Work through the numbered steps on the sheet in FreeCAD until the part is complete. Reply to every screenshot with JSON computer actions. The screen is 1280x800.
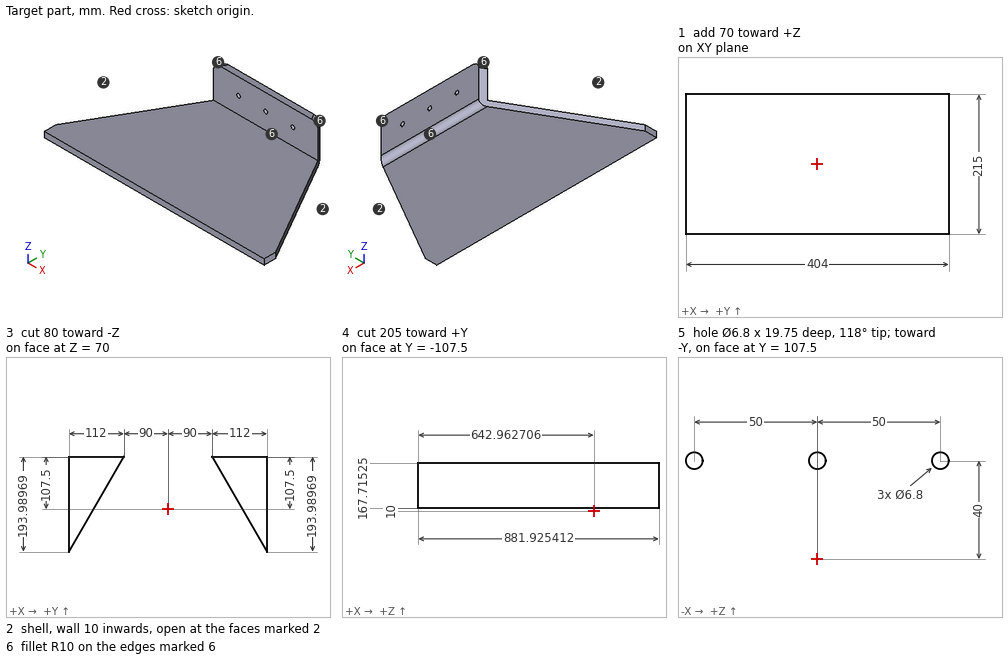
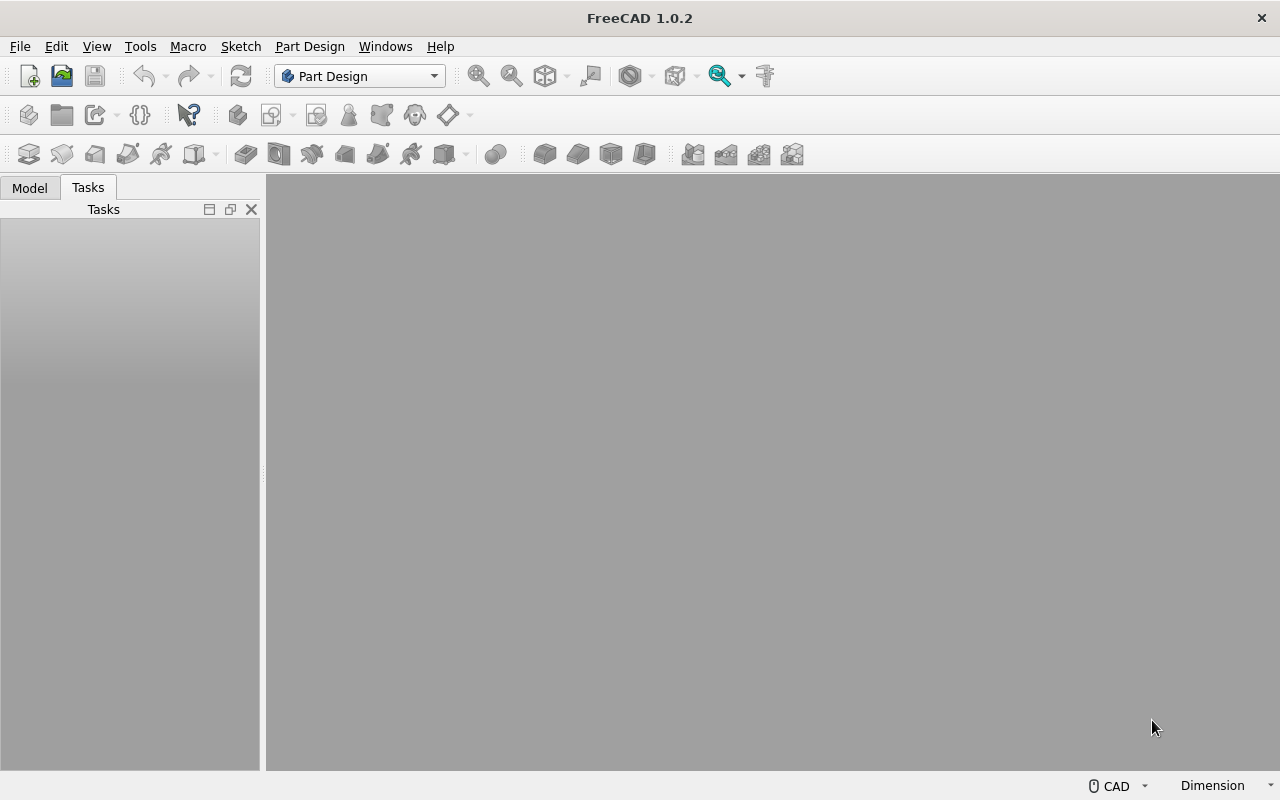
{"action": "left_click", "coordinate": [29, 76]}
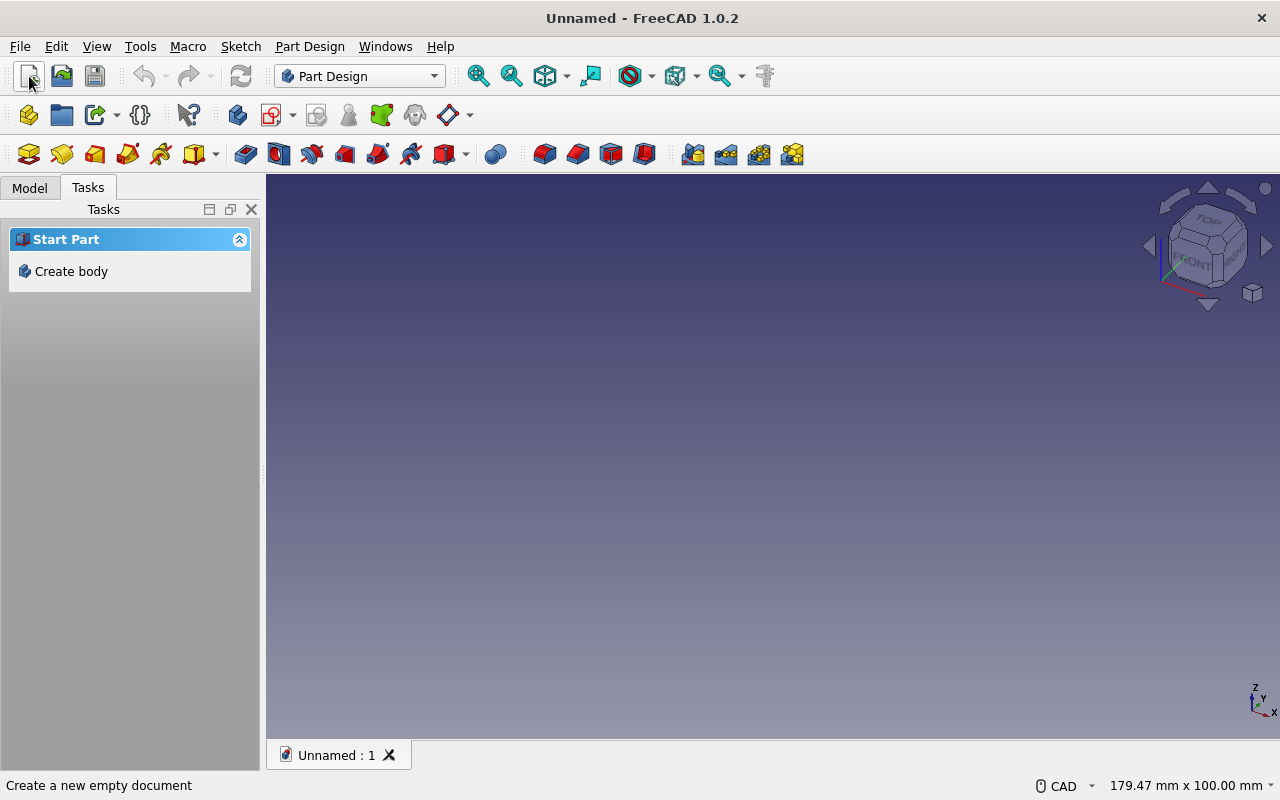
{"action": "left_click", "coordinate": [270, 116]}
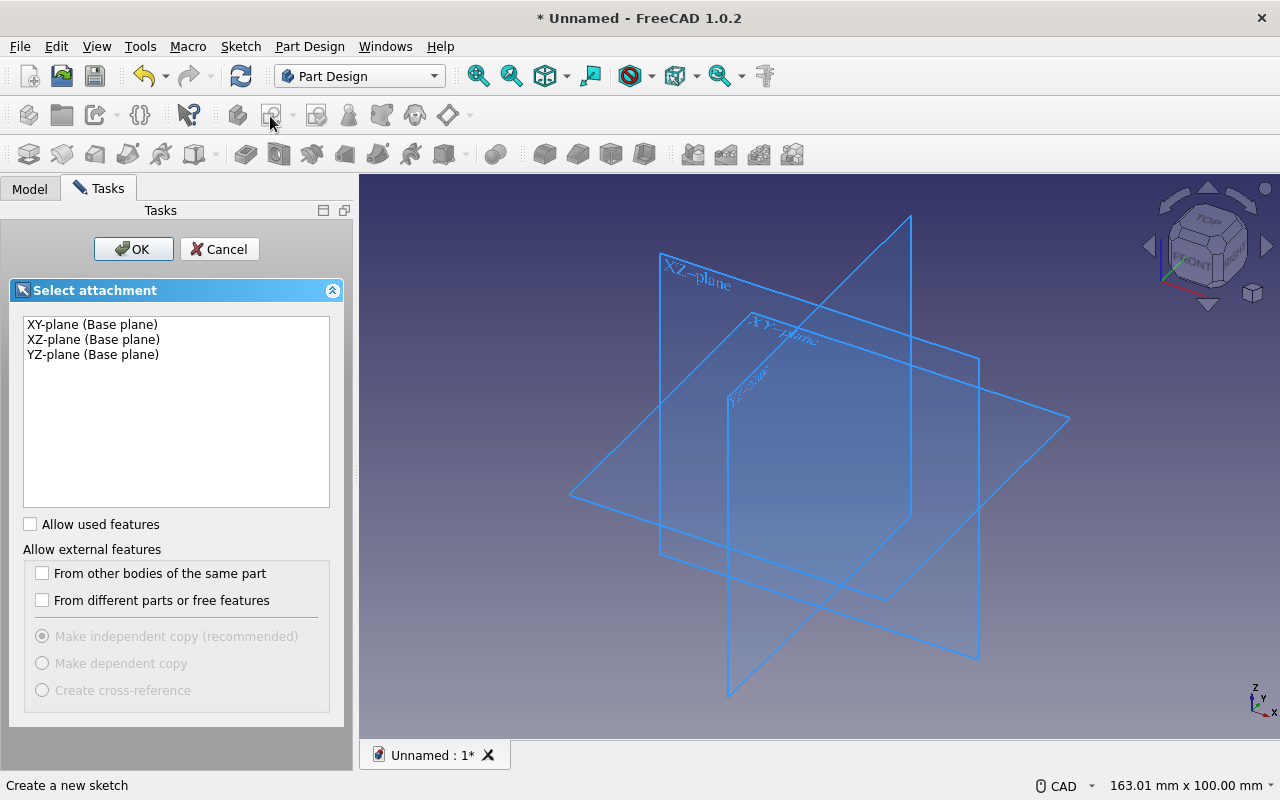
{"action": "left_click", "coordinate": [84, 324]}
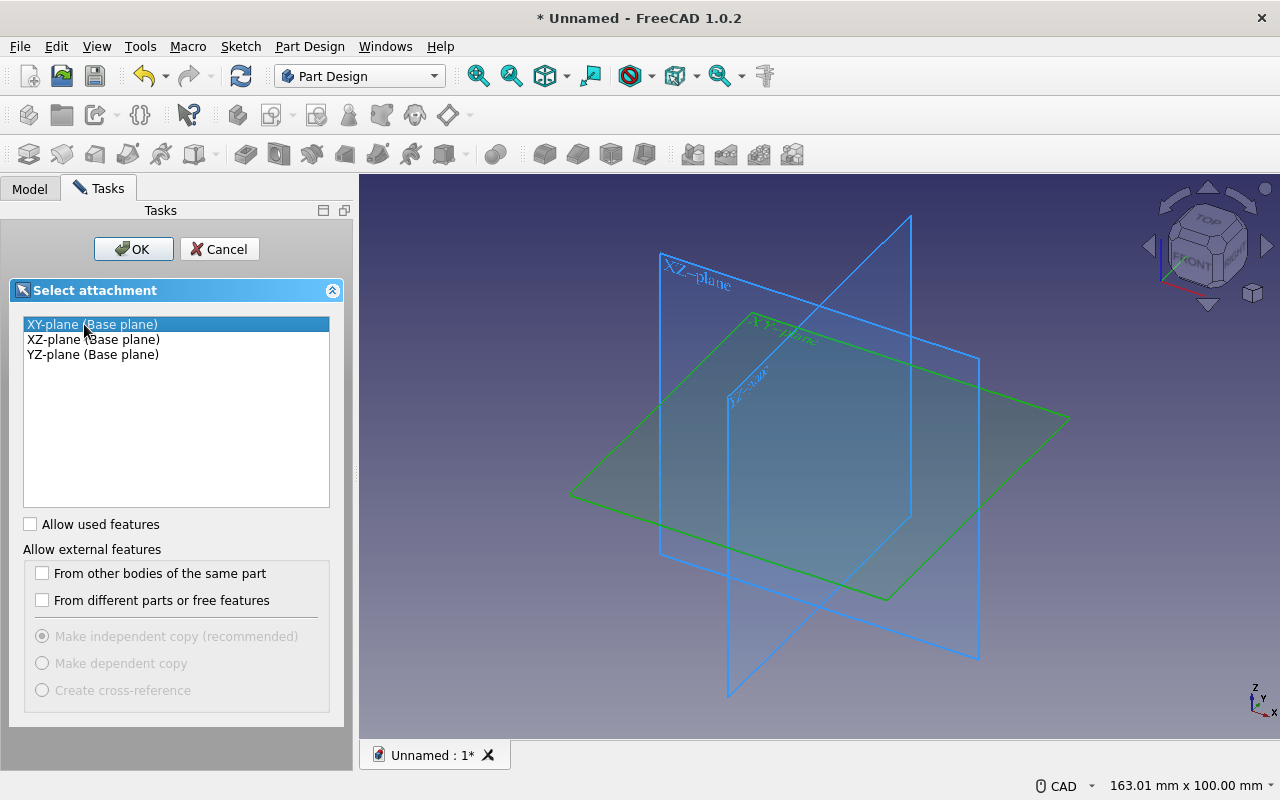
{"action": "left_click", "coordinate": [134, 249]}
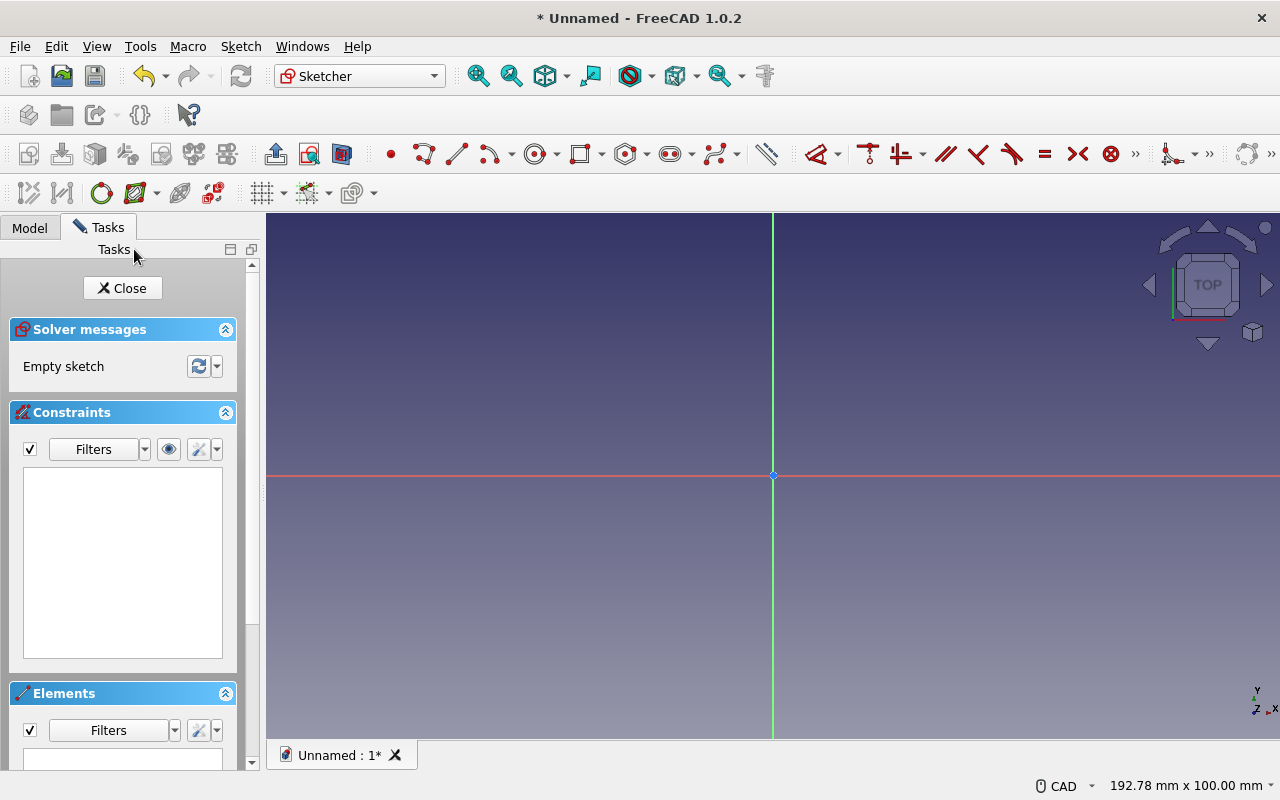
{"action": "scroll", "coordinate": [675, 476], "scroll_direction": "down", "scroll_amount": 6}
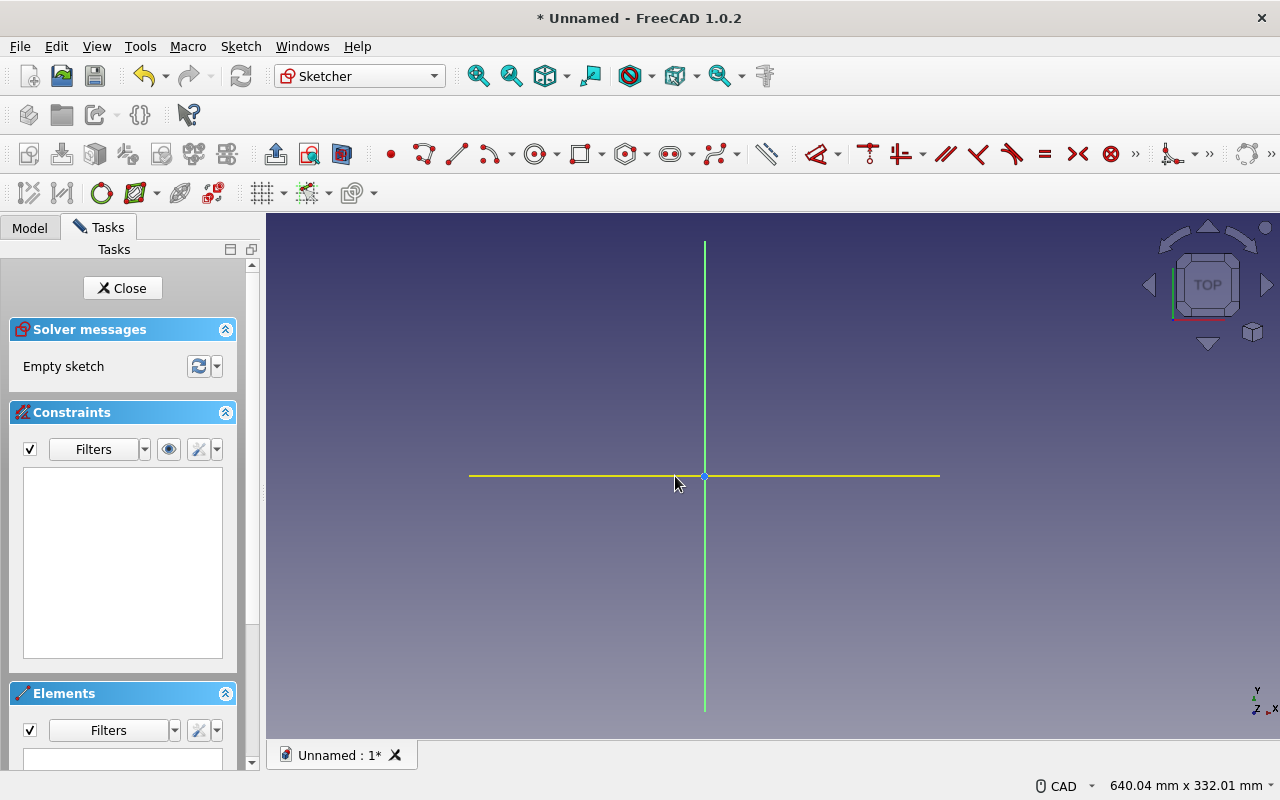
{"action": "key", "text": "g v"}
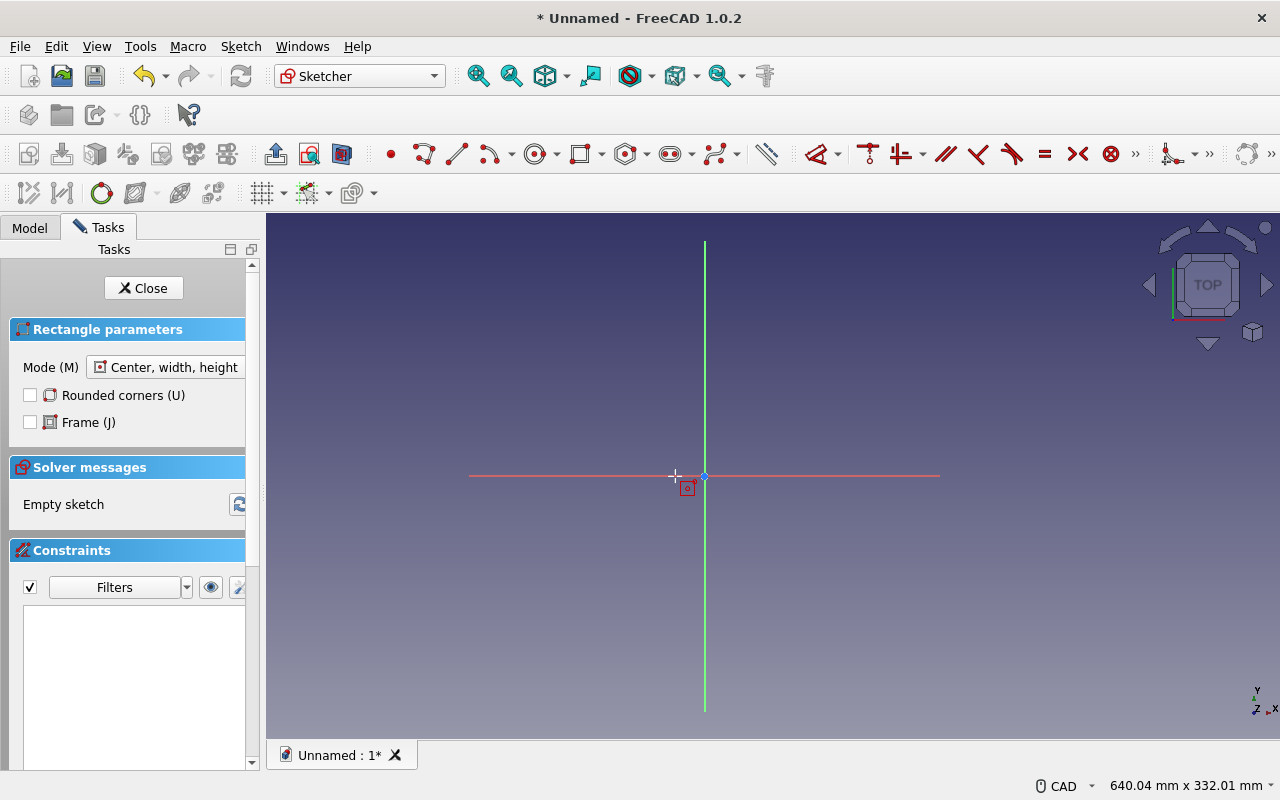
{"action": "left_click", "coordinate": [705, 476]}
{"action": "left_click", "coordinate": [1025, 306]}
{"action": "key", "text": "Escape"}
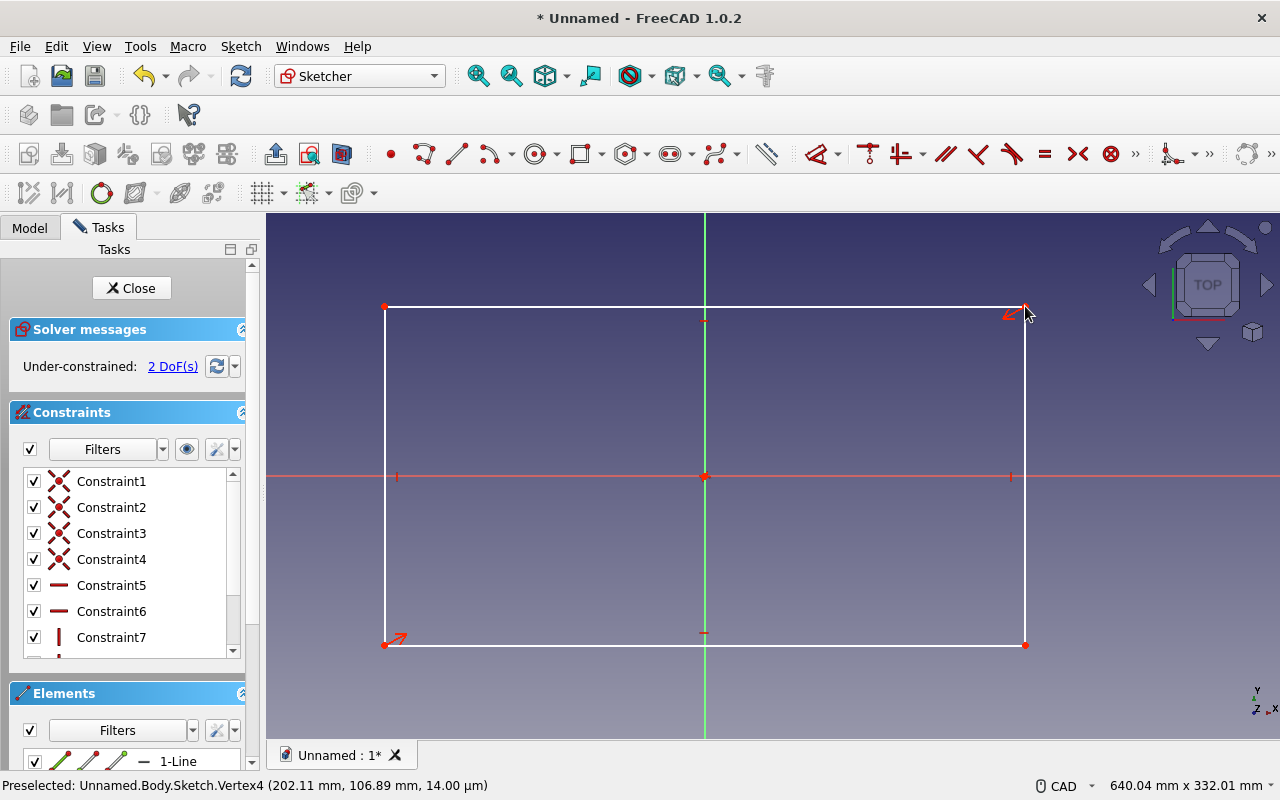
{"action": "left_click", "coordinate": [577, 646]}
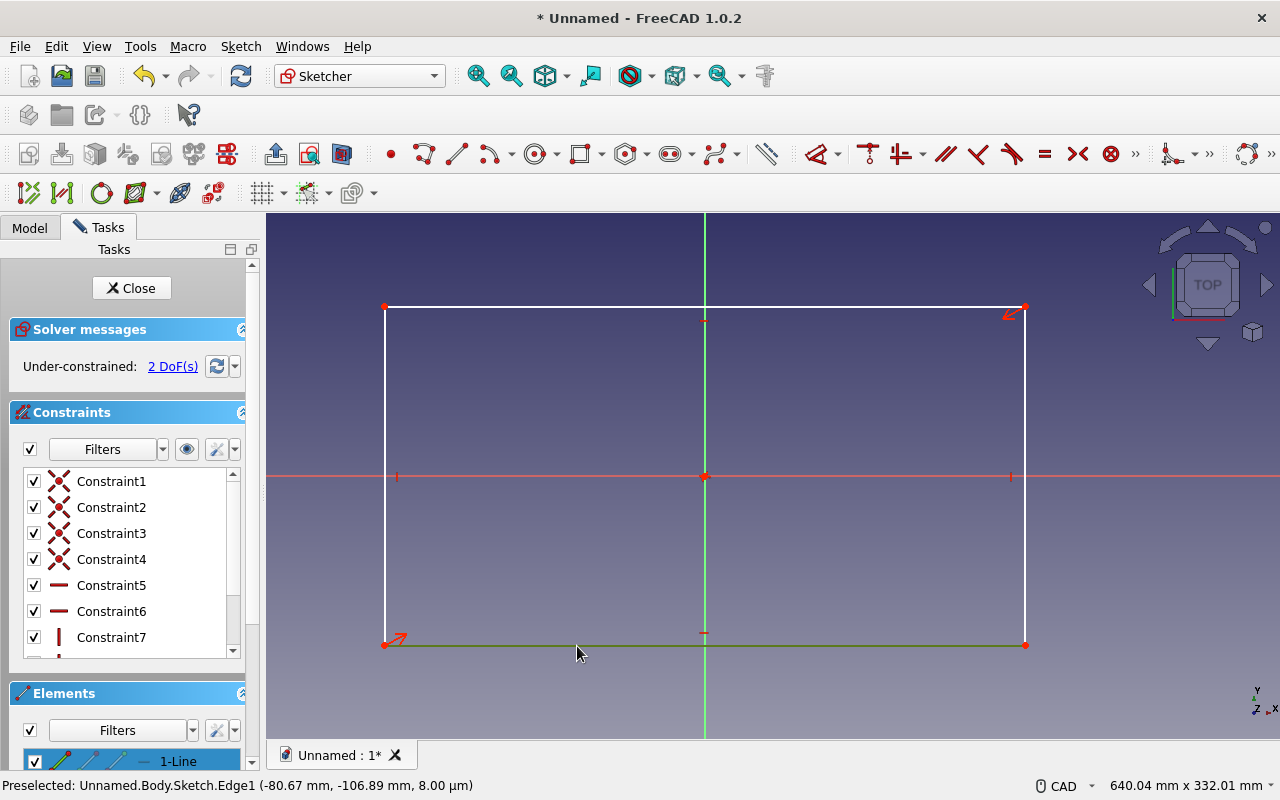
{"action": "left_click", "coordinate": [838, 154]}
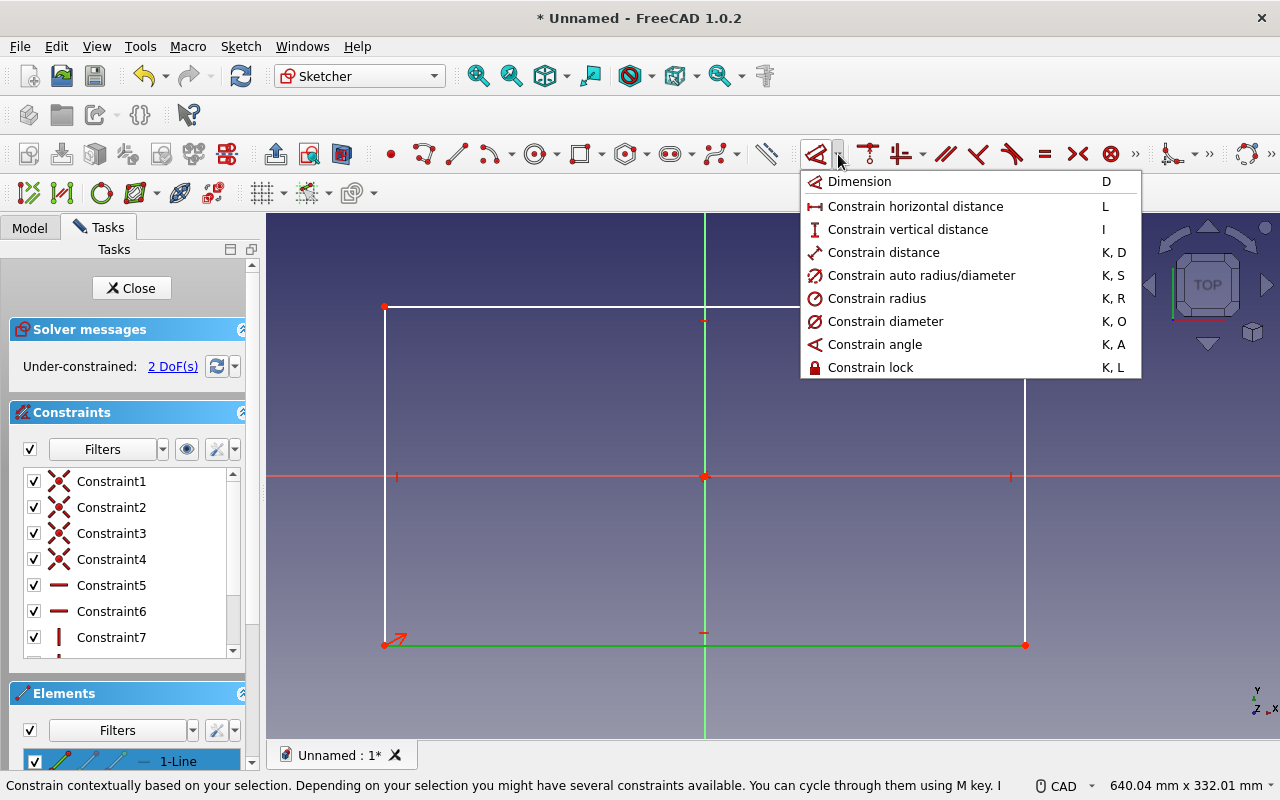
{"action": "left_click", "coordinate": [971, 206]}